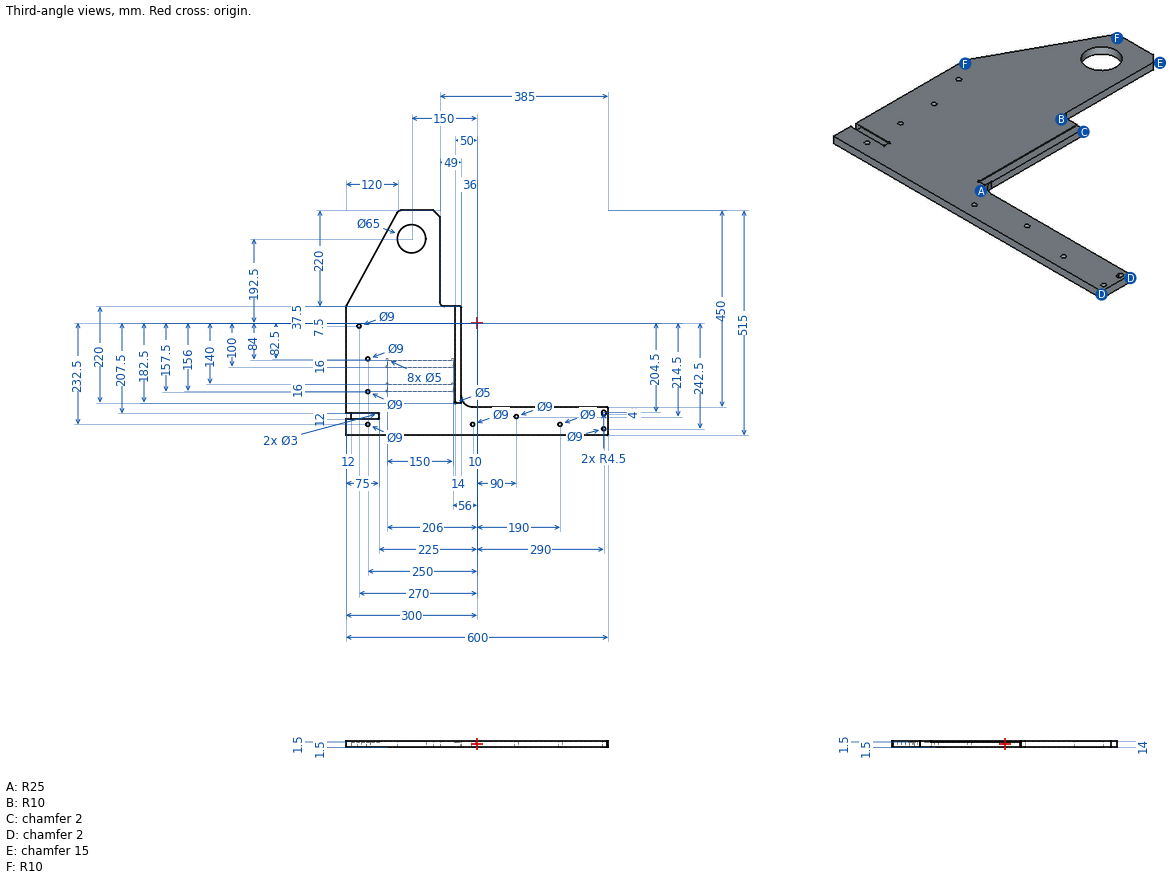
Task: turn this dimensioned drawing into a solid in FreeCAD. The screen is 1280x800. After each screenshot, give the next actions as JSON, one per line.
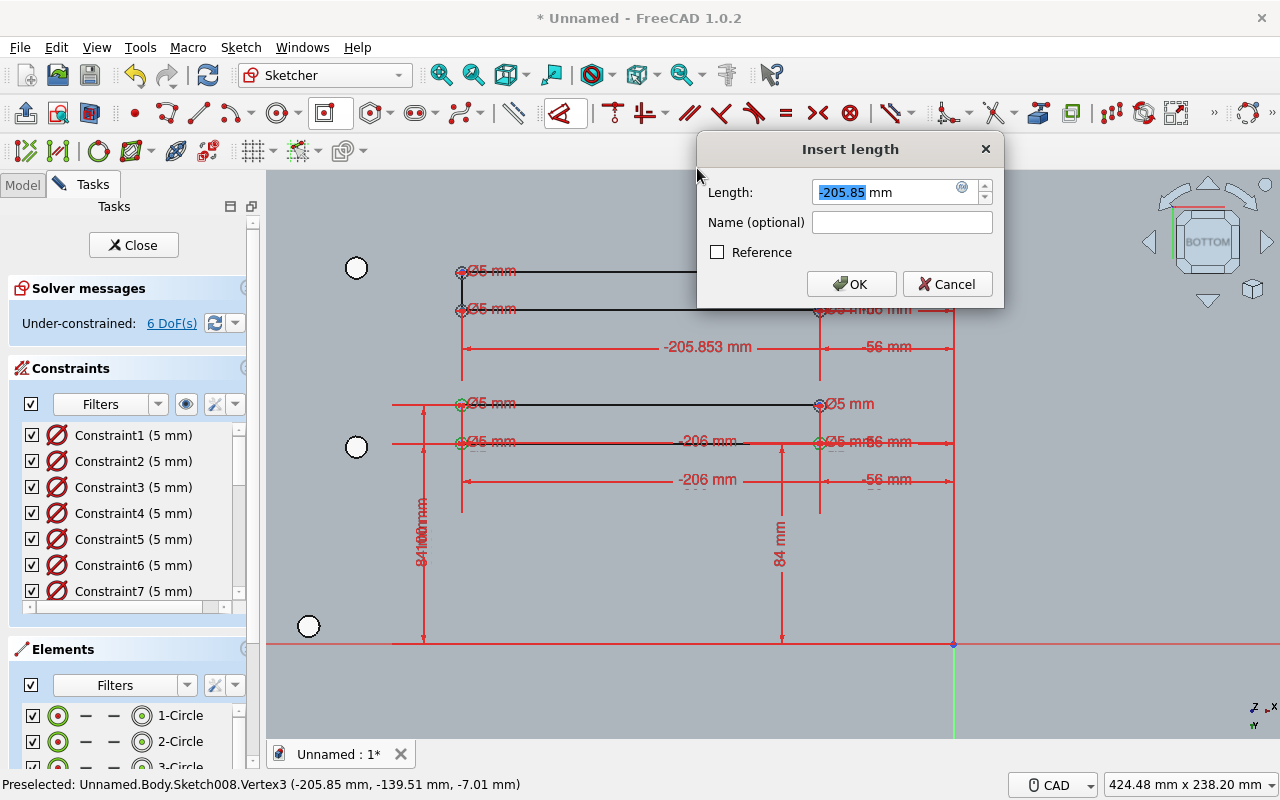
{"action": "type", "text": "-206"}
{"action": "key", "text": "Return"}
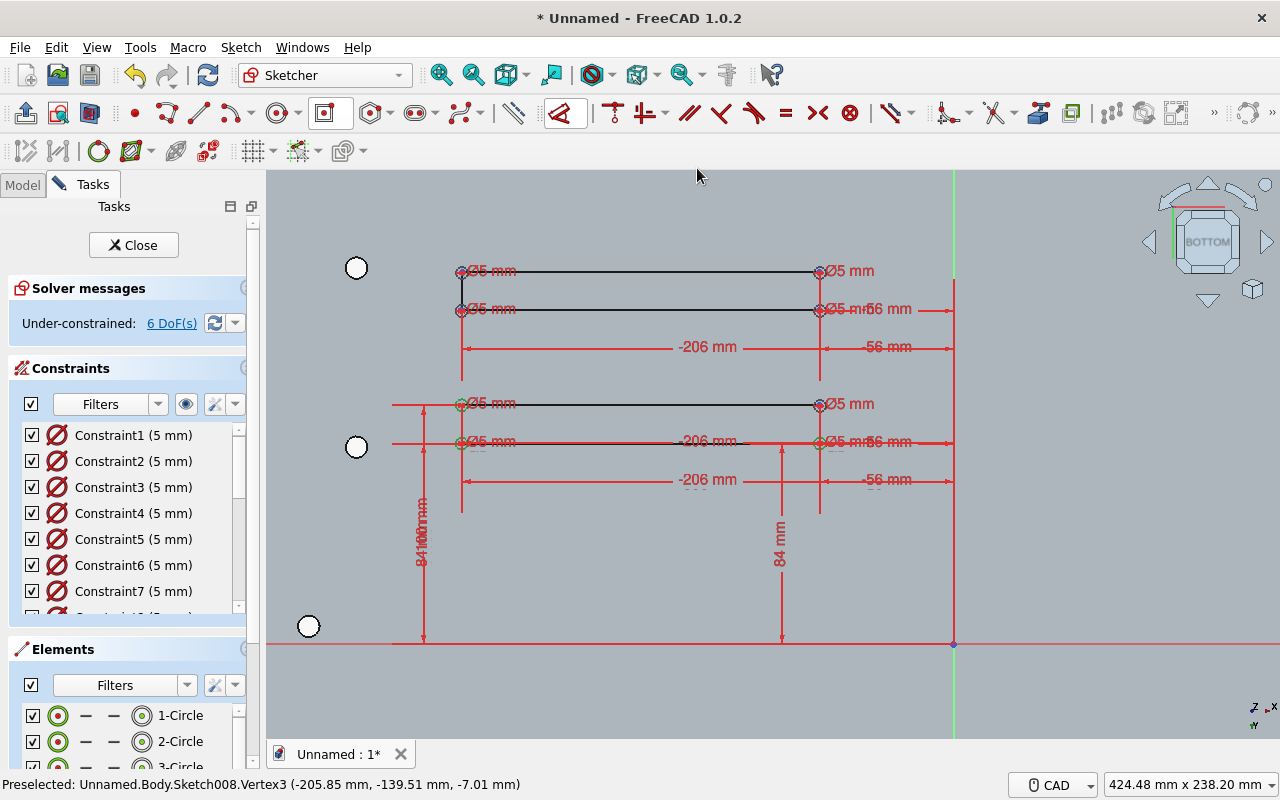
{"action": "left_click", "coordinate": [462, 311]}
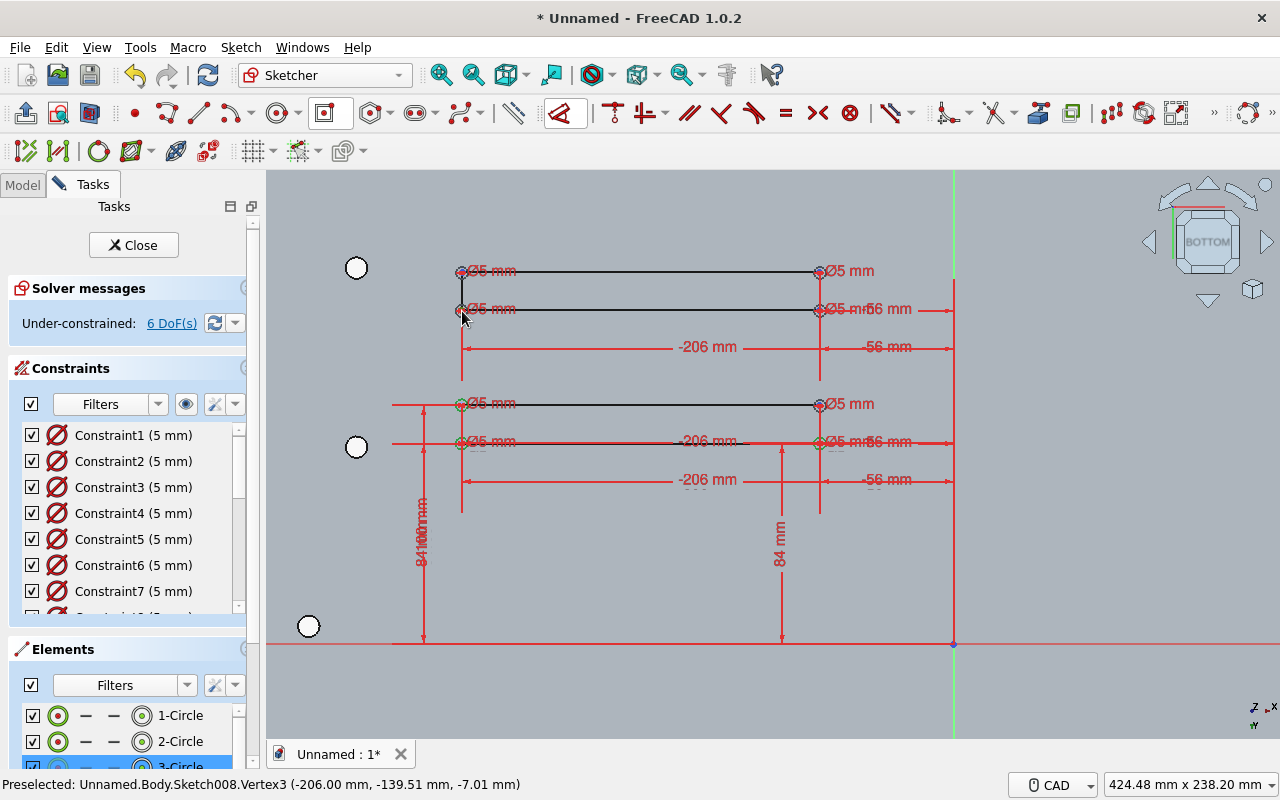
{"action": "left_click", "coordinate": [582, 114]}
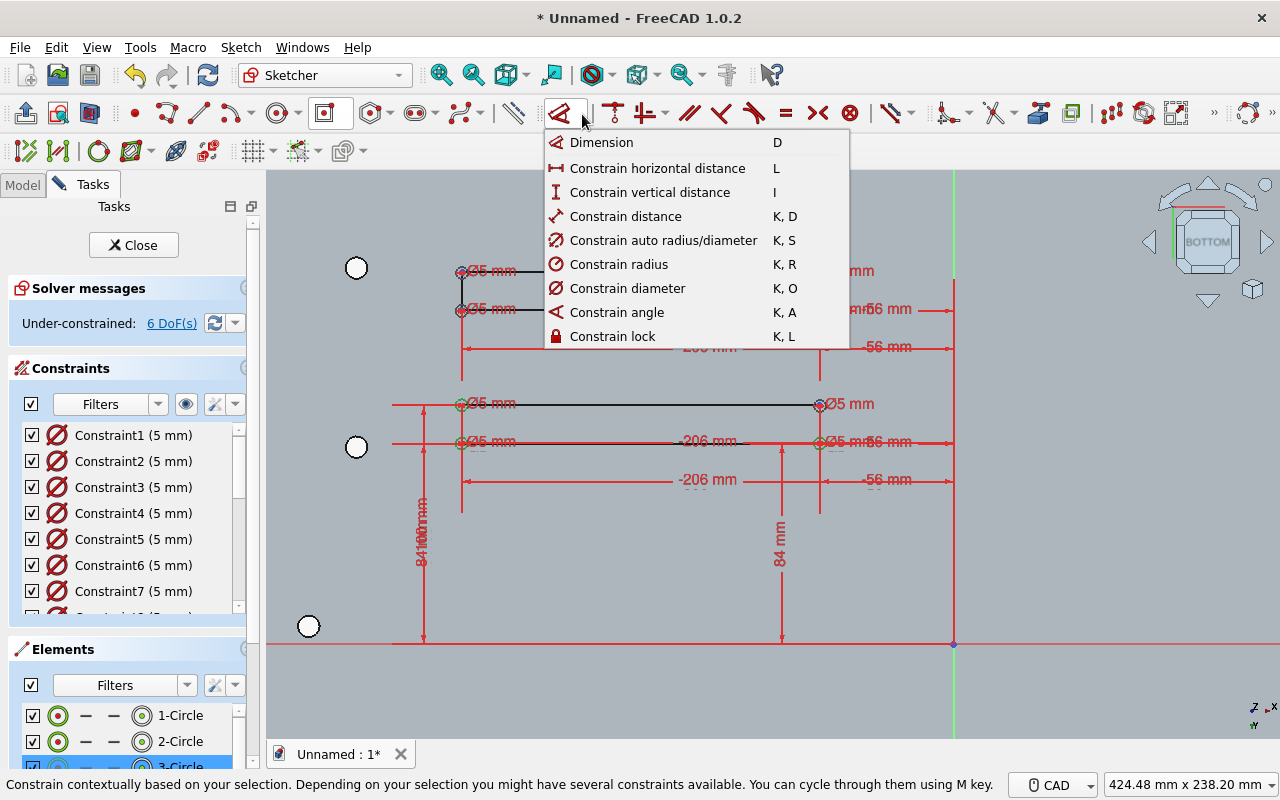
{"action": "left_click", "coordinate": [697, 192]}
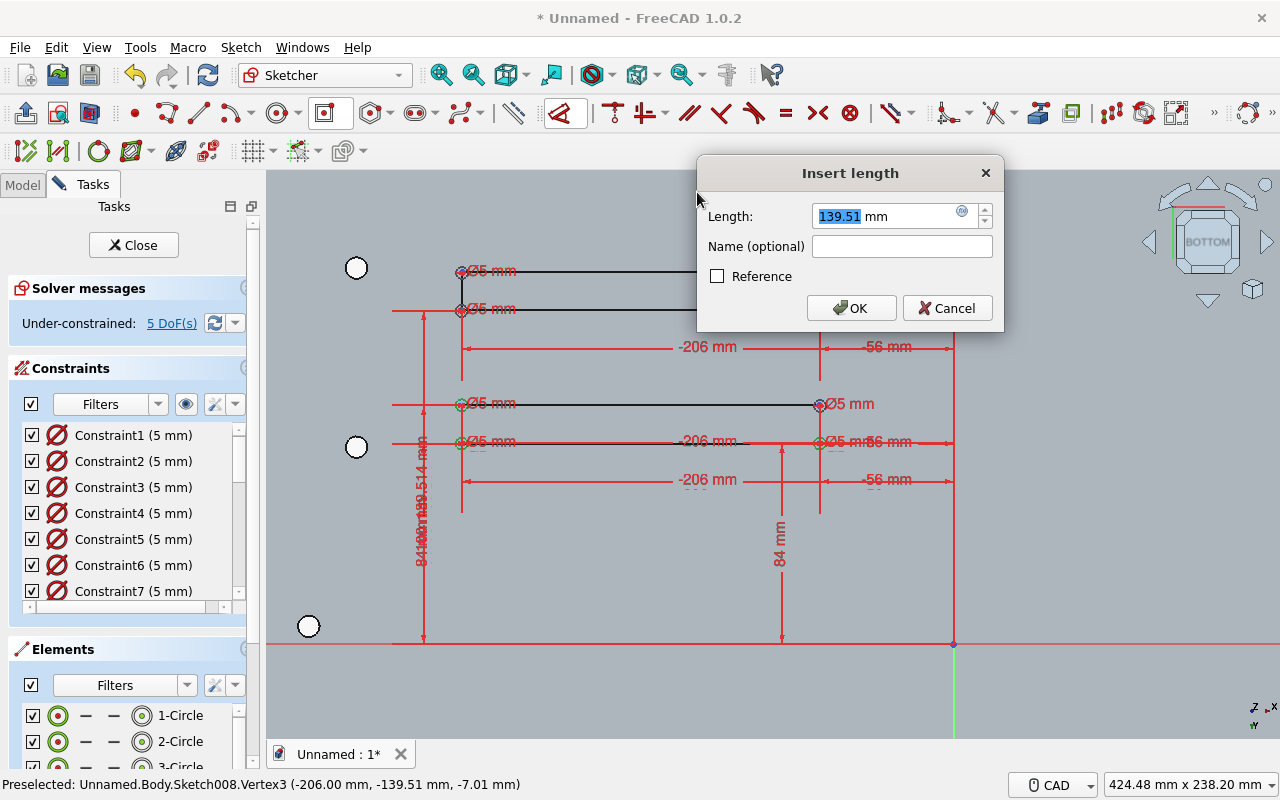
{"action": "type", "text": "140"}
{"action": "key", "text": "Return"}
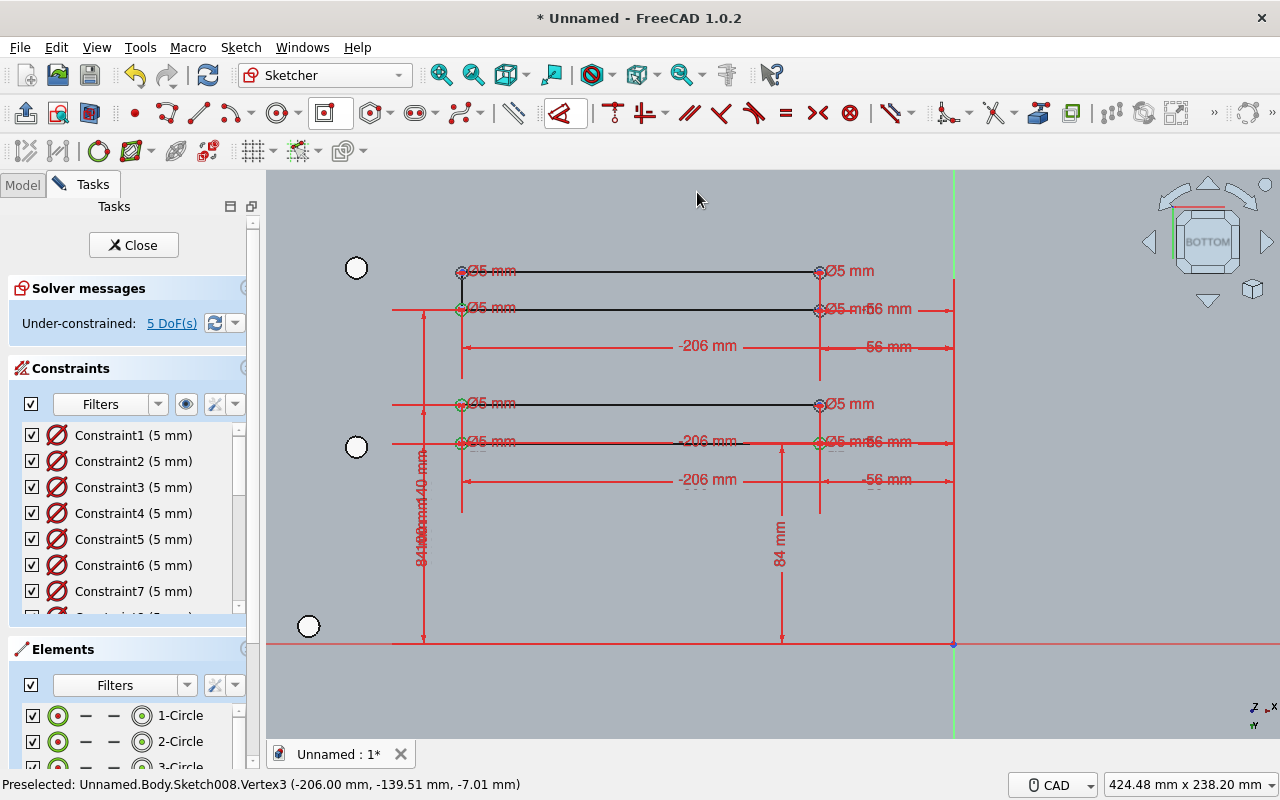
{"action": "left_click", "coordinate": [462, 273]}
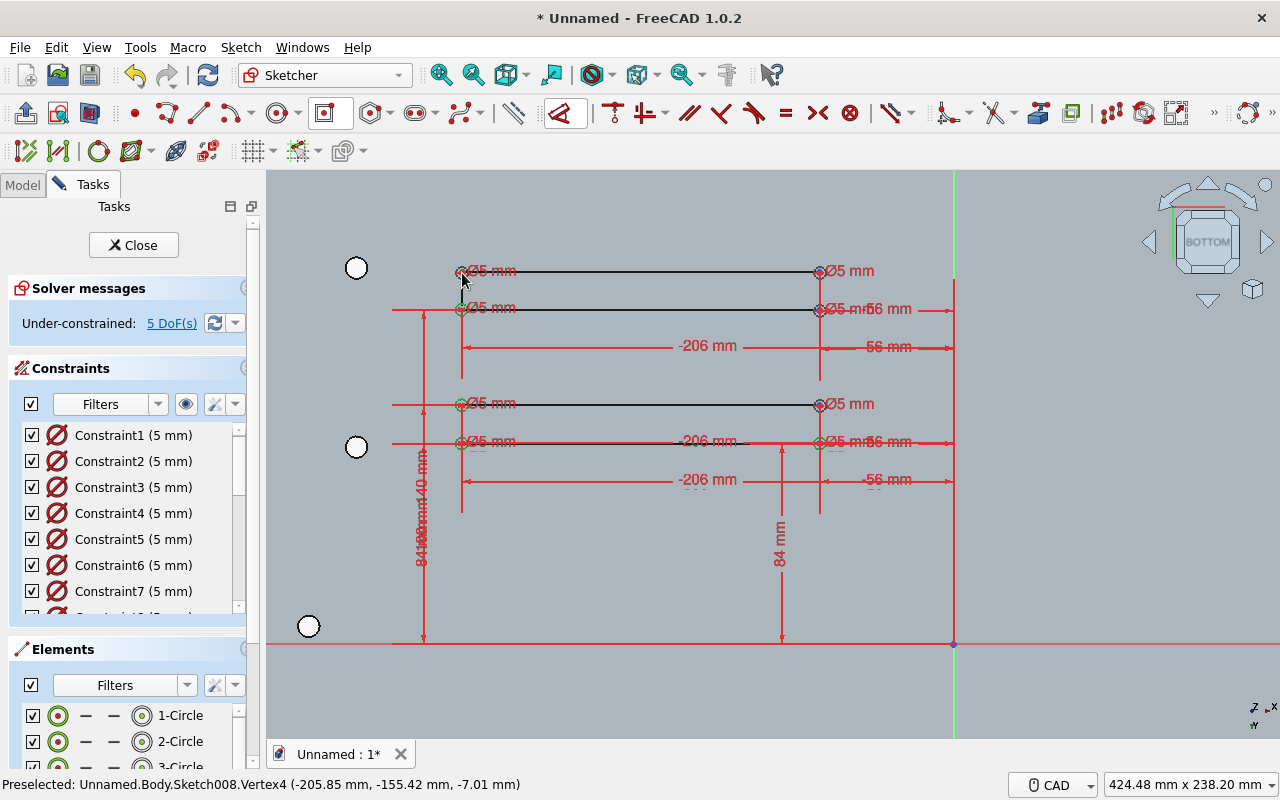
{"action": "left_click", "coordinate": [582, 114]}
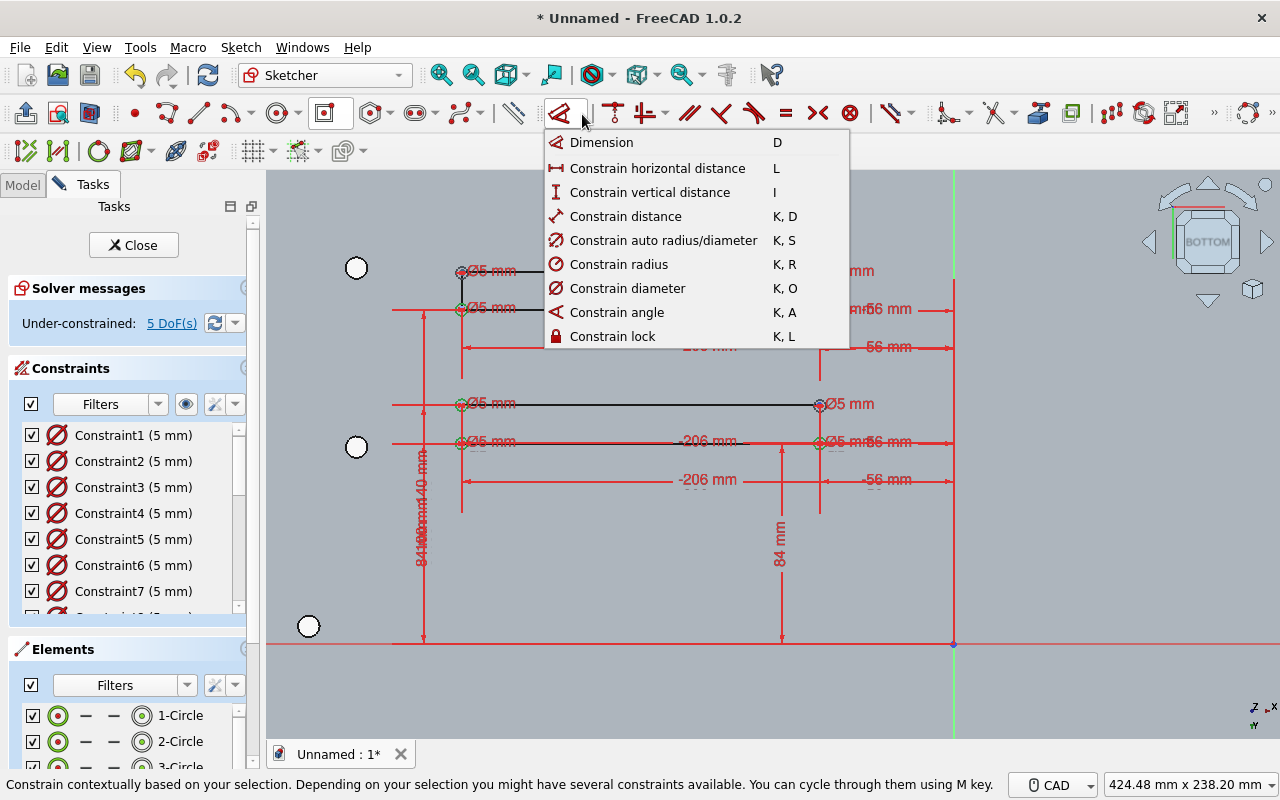
{"action": "left_click", "coordinate": [697, 168]}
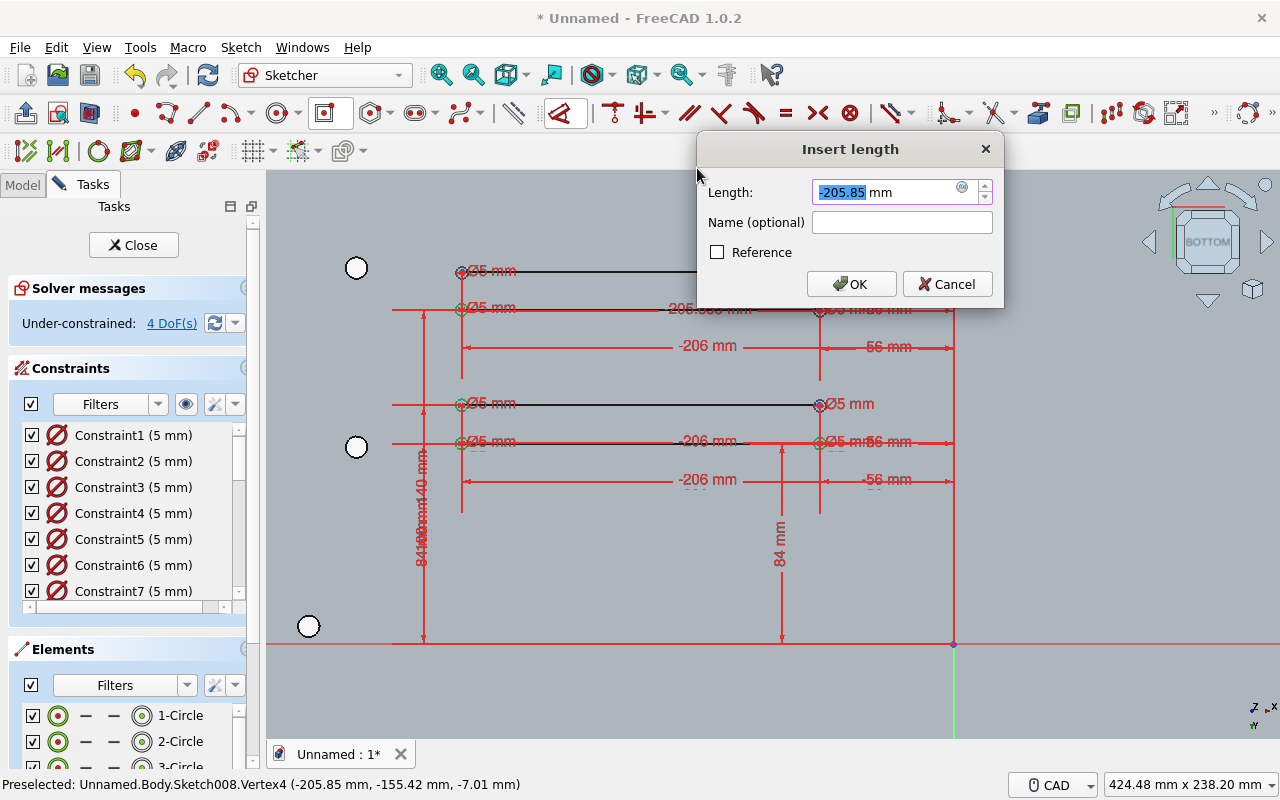
{"action": "type", "text": "-206"}
{"action": "key", "text": "Return"}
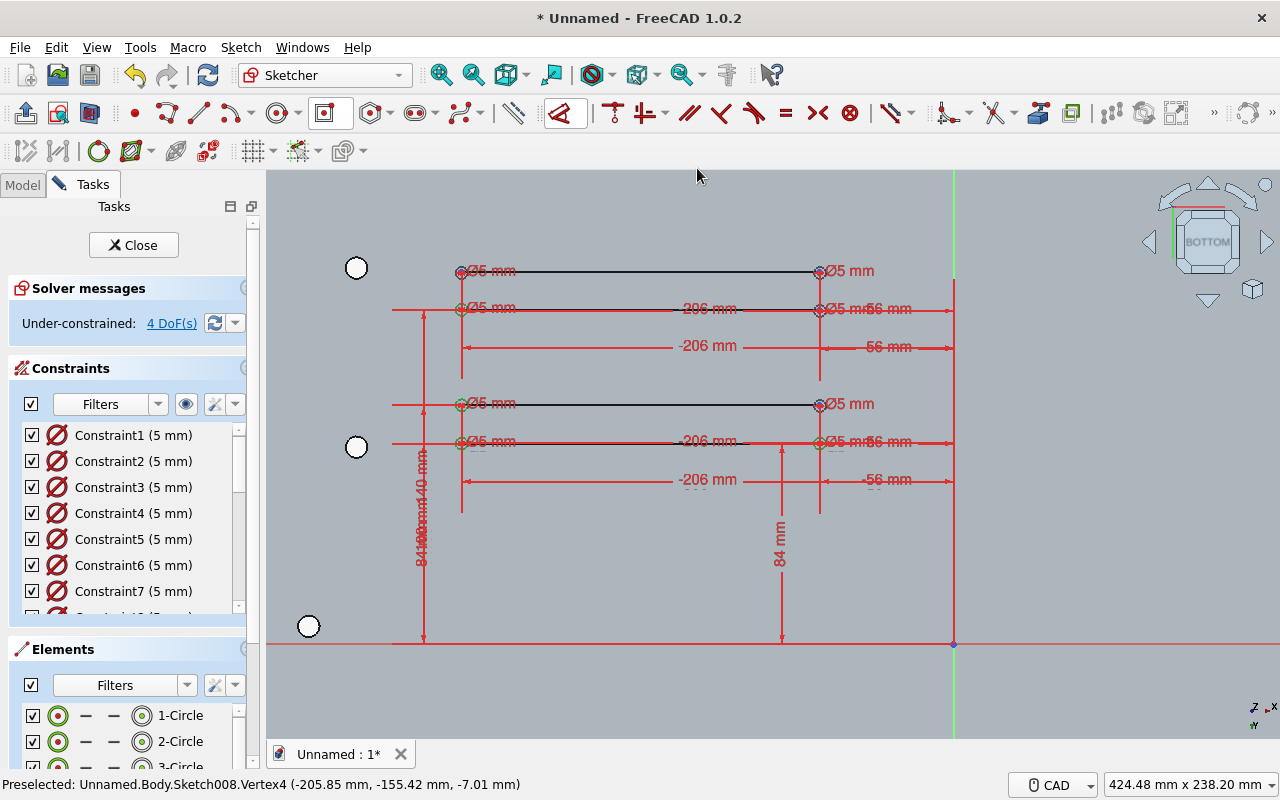
{"action": "left_click", "coordinate": [462, 273]}